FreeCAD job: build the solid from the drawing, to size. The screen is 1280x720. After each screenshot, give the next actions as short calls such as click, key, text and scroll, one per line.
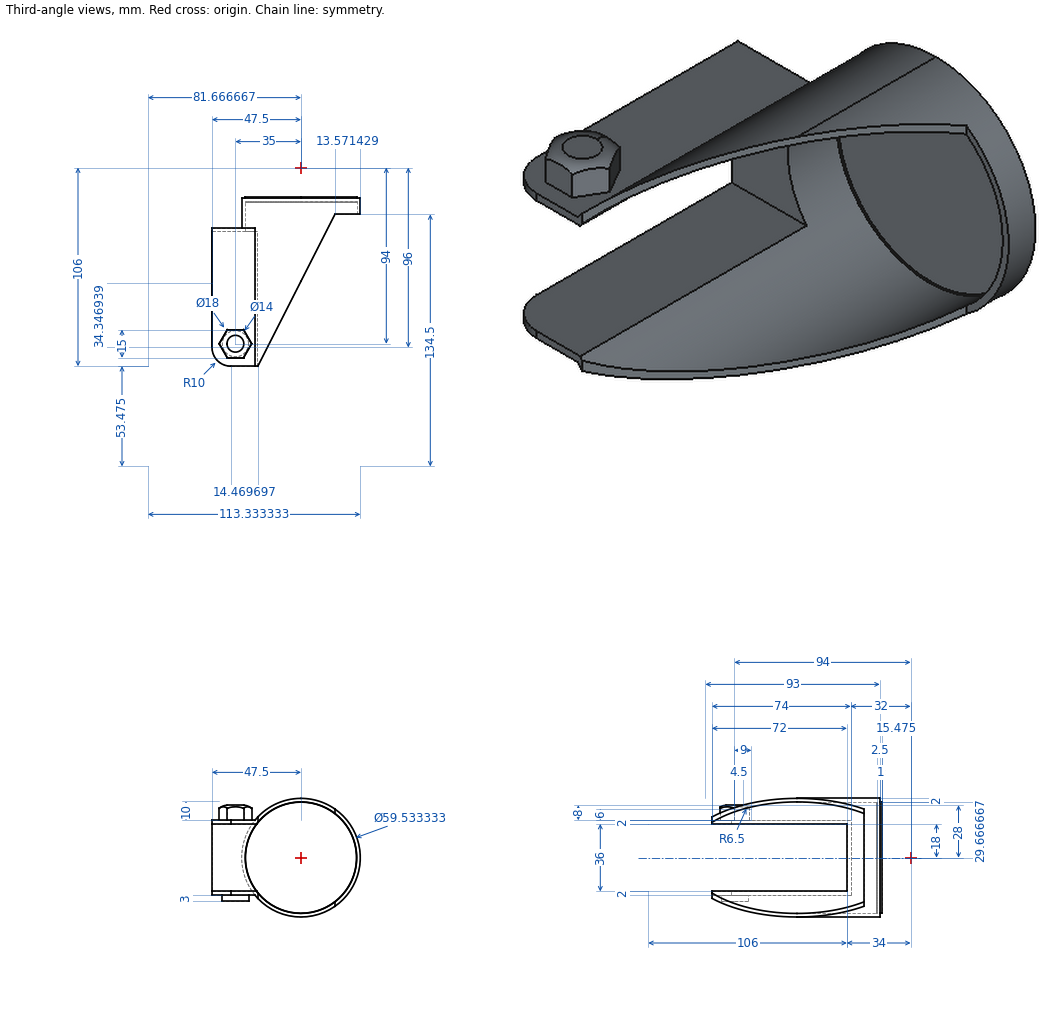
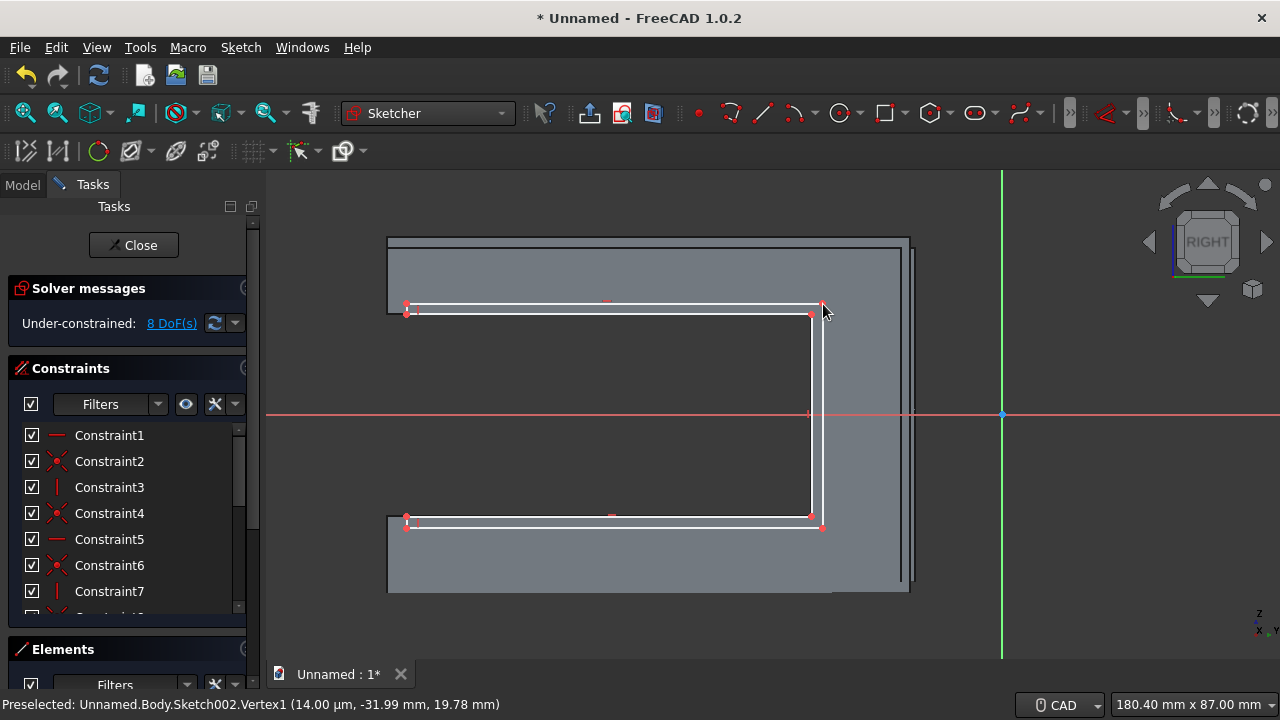
click(407, 314)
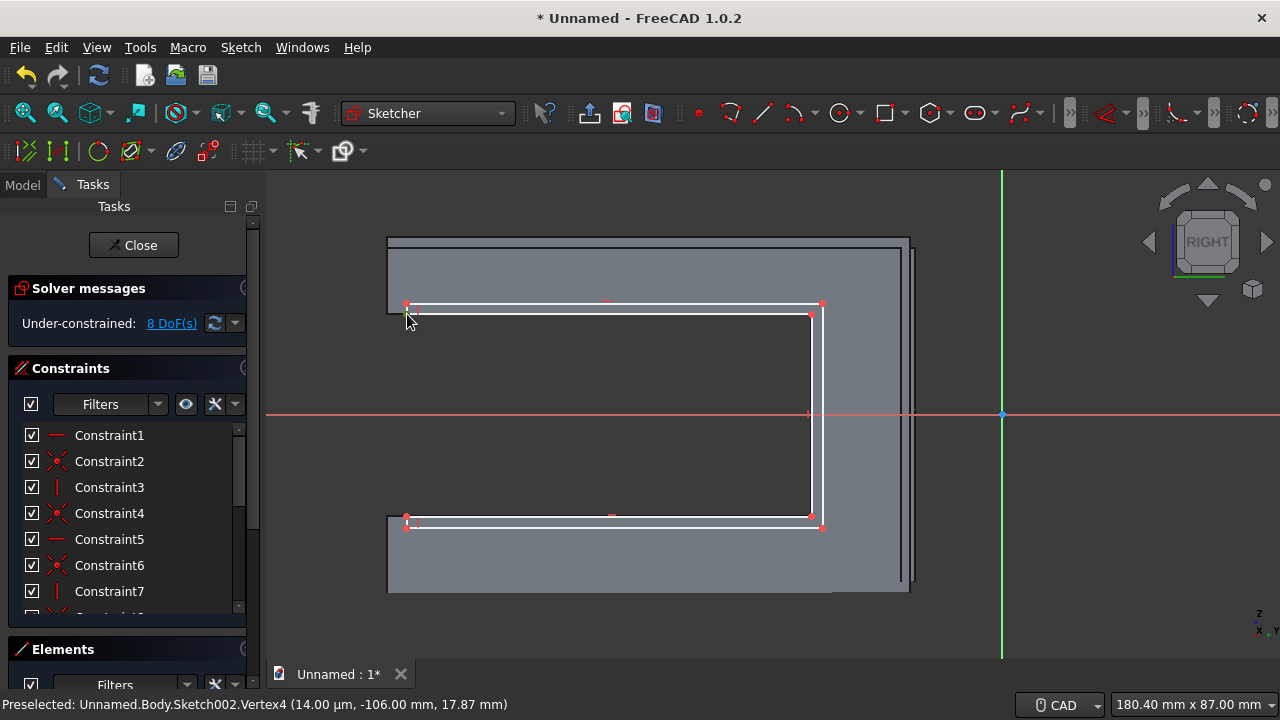
click(407, 517)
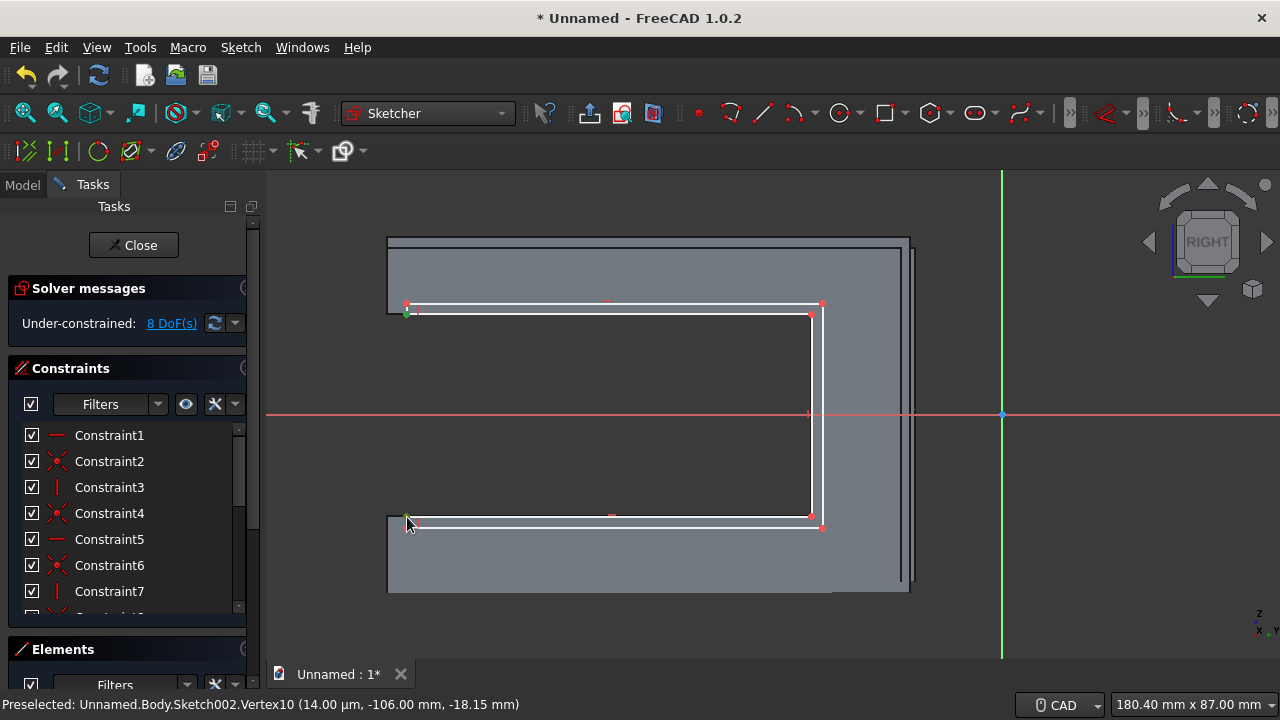
click(353, 415)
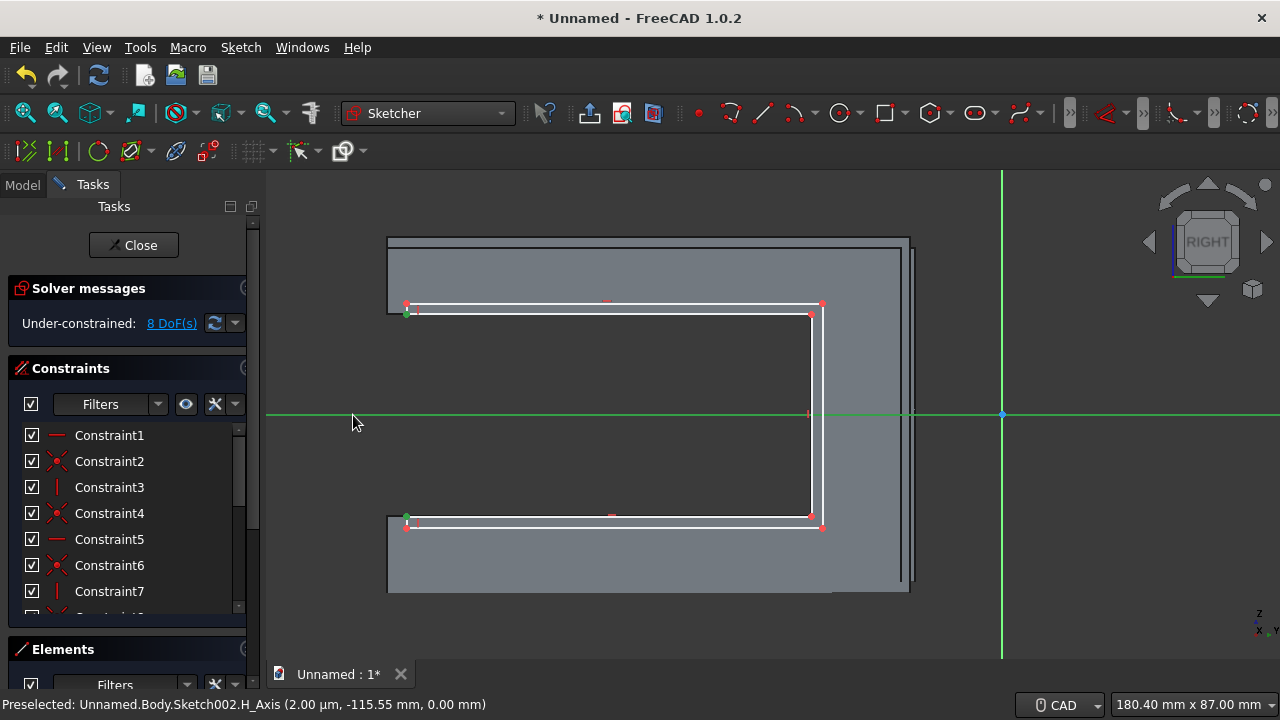
key(s)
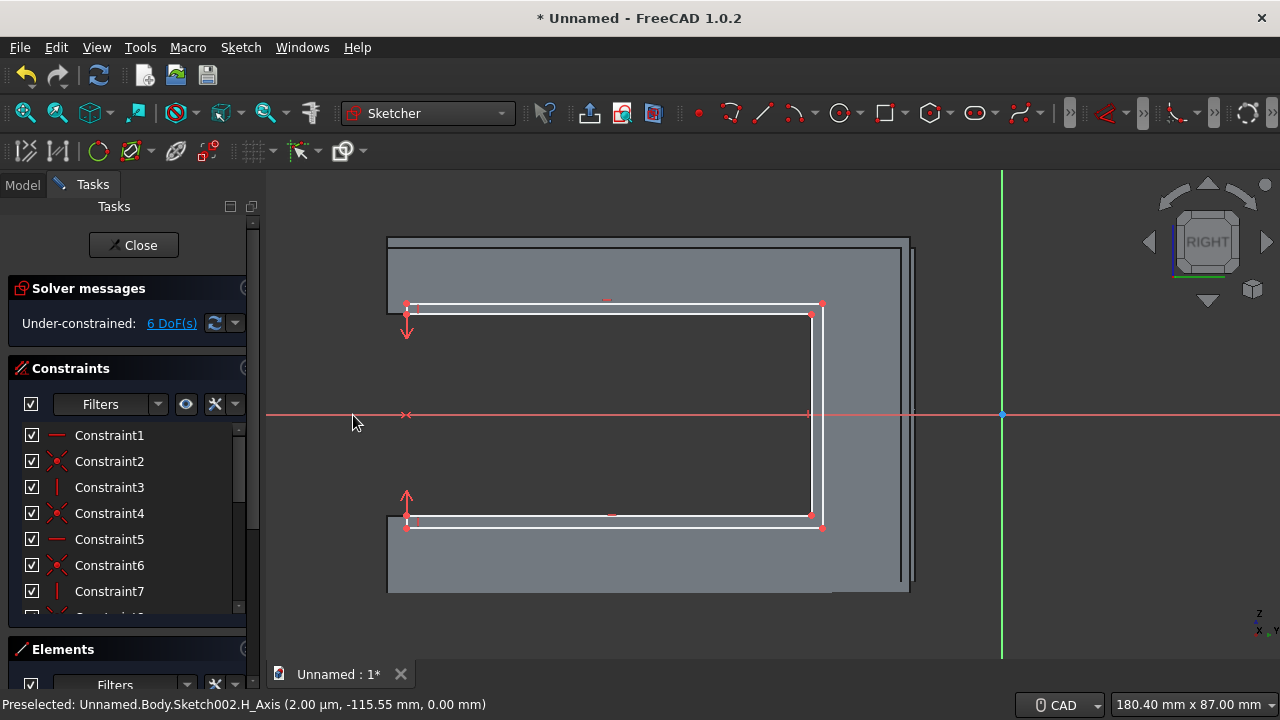
key(d)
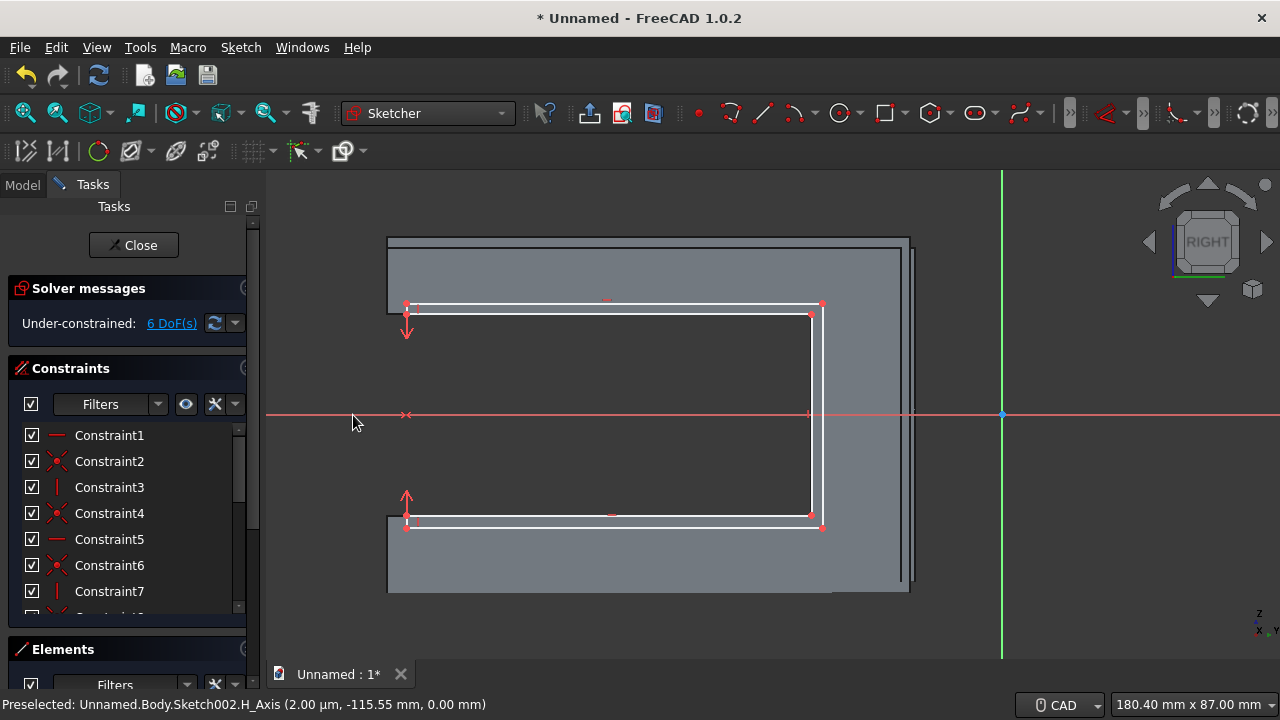
scroll(407, 309, up, 7)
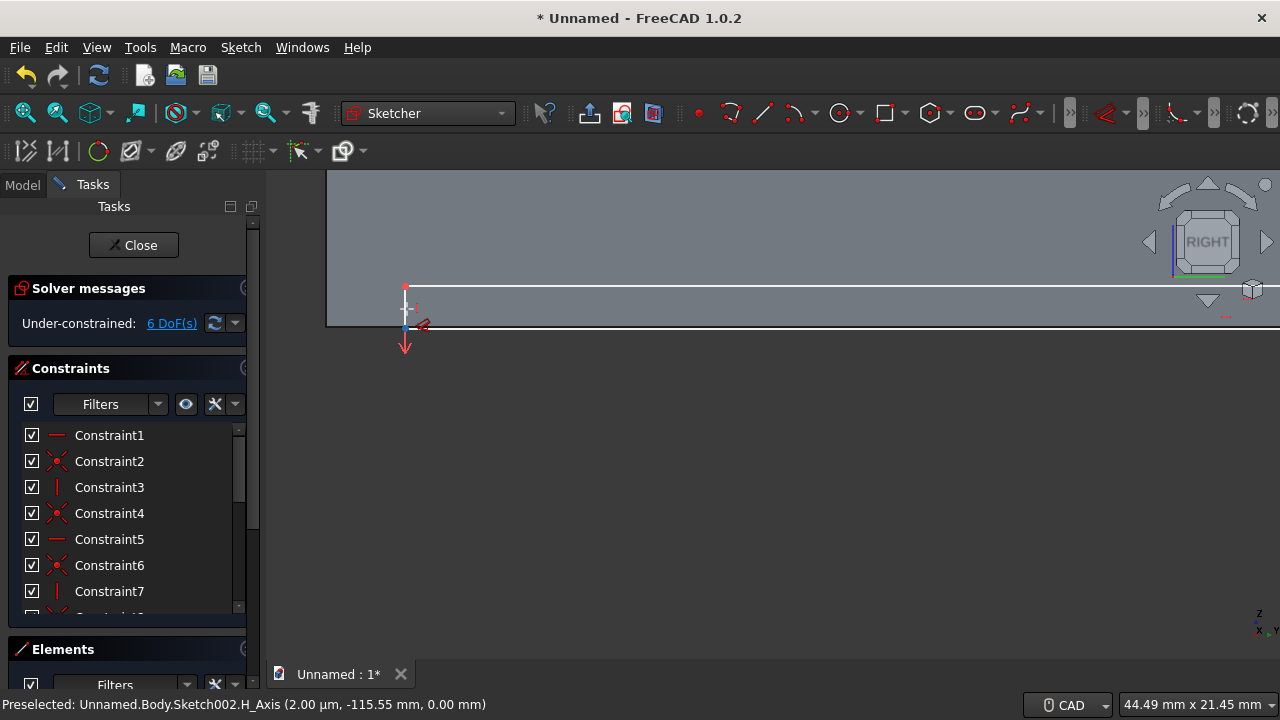
click(405, 308)
click(371, 308)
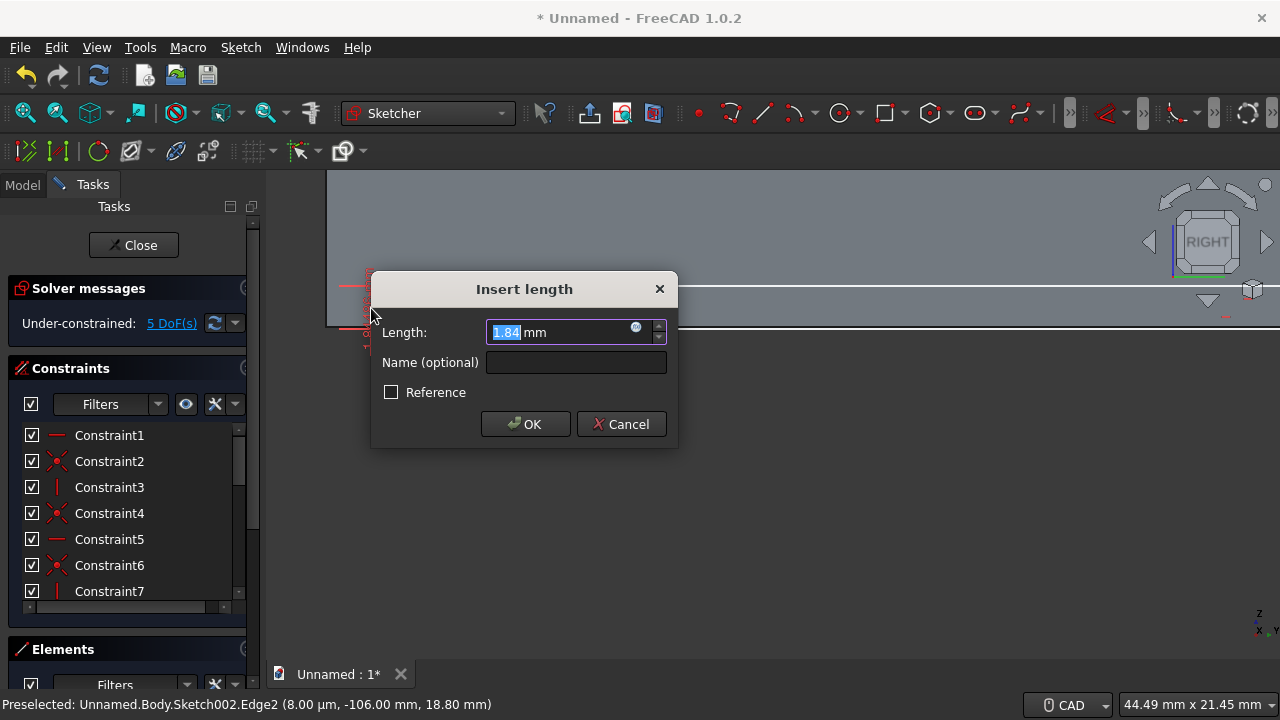
text(2)
key(Return)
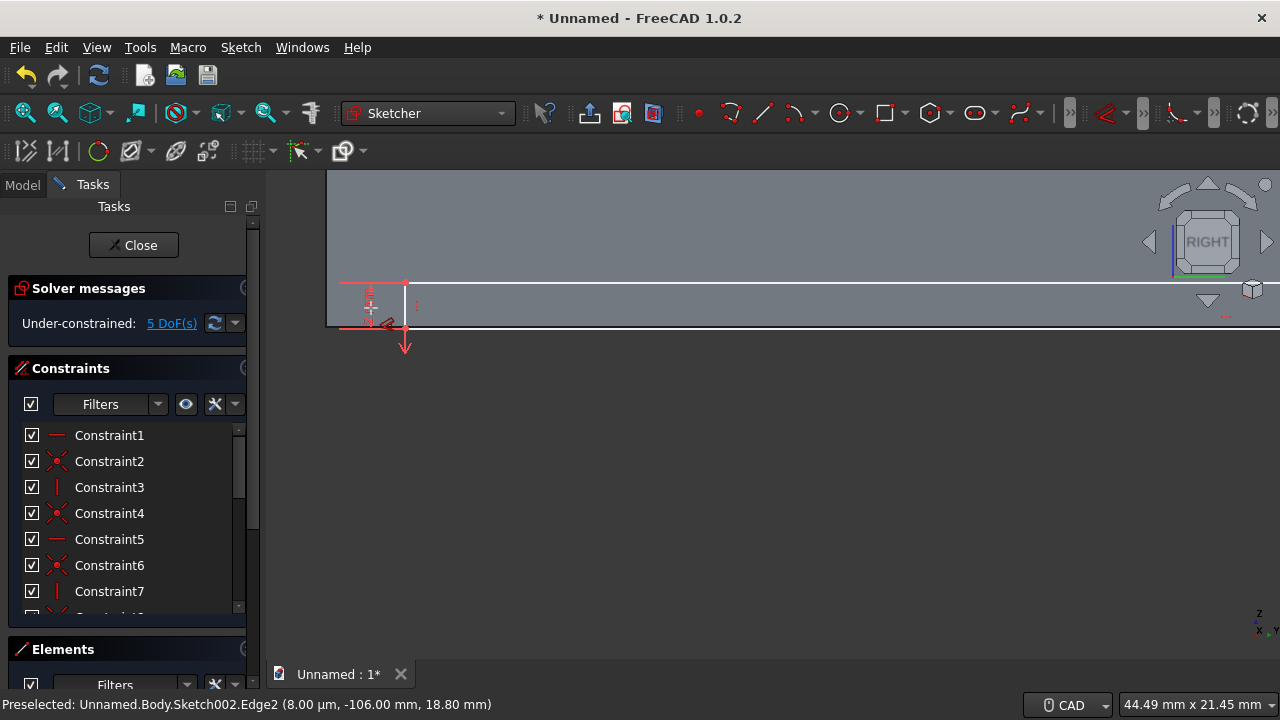
scroll(407, 309, down, 7)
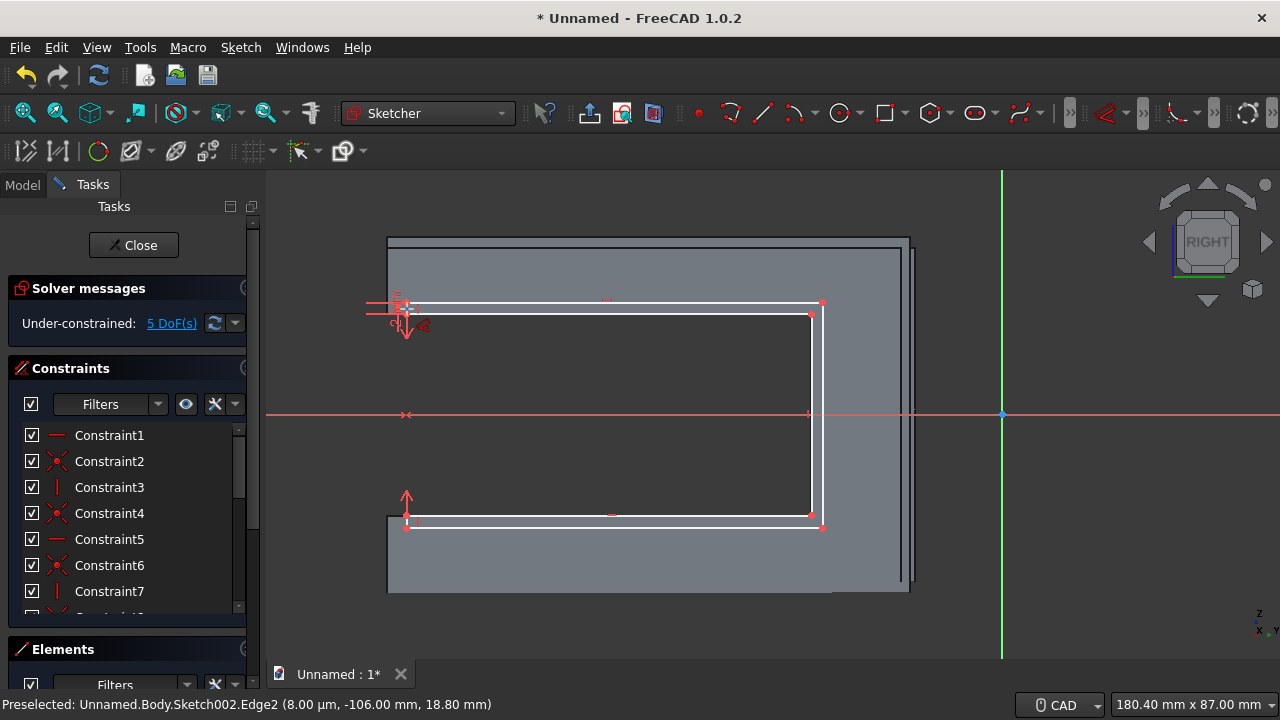
scroll(407, 519, up, 7)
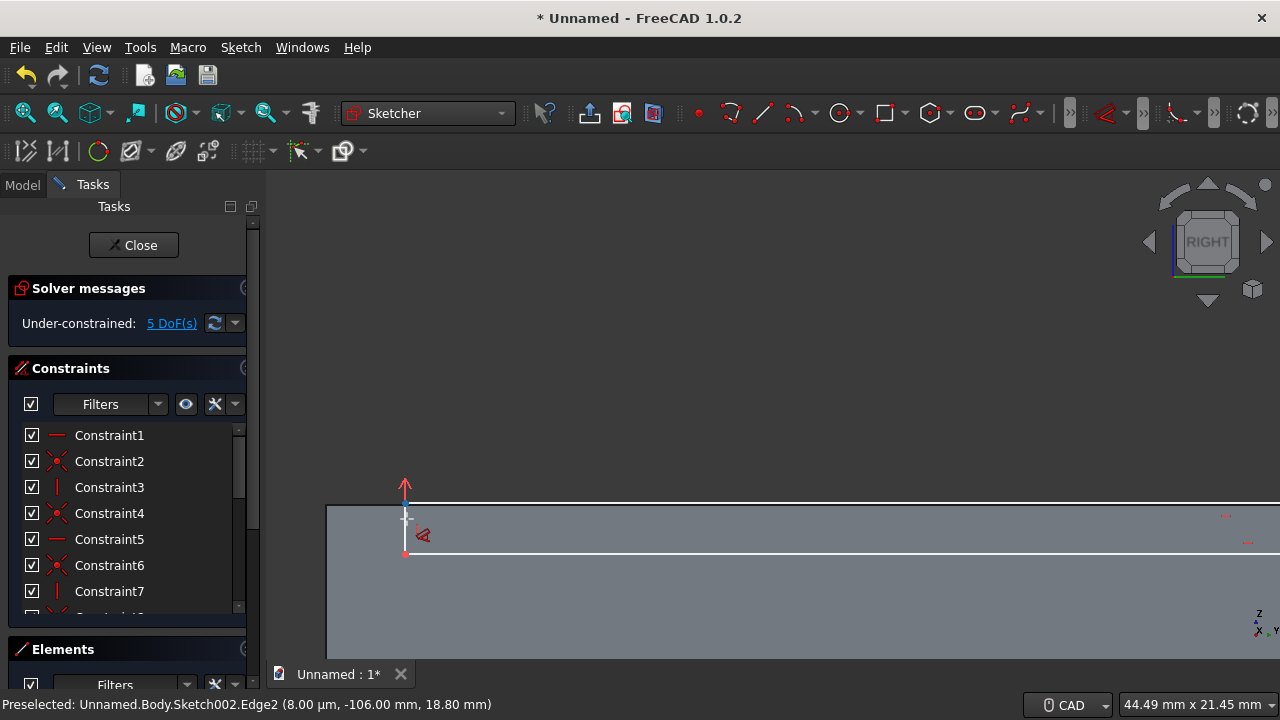
click(405, 519)
click(371, 529)